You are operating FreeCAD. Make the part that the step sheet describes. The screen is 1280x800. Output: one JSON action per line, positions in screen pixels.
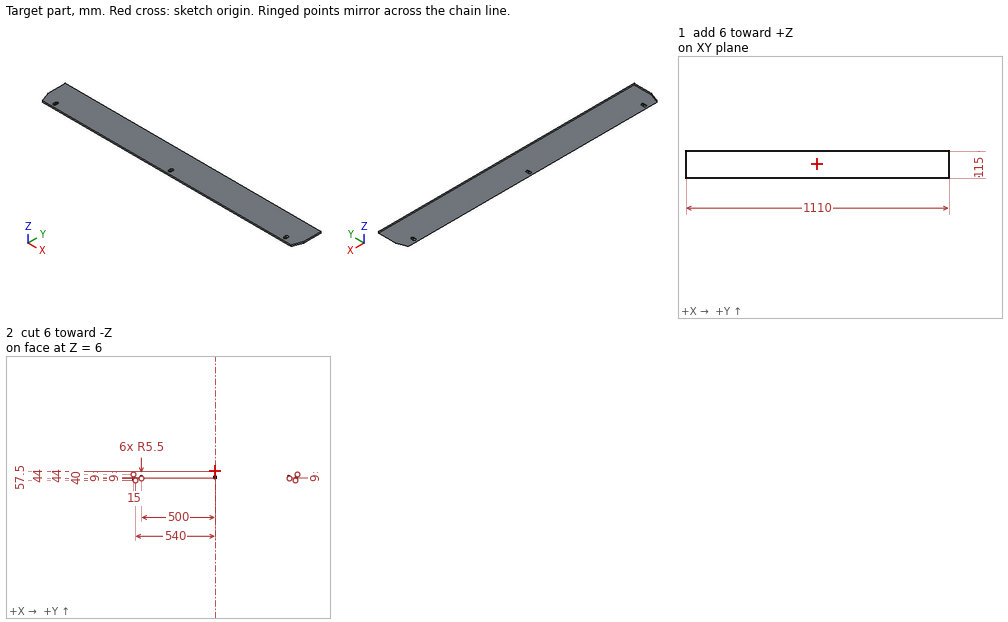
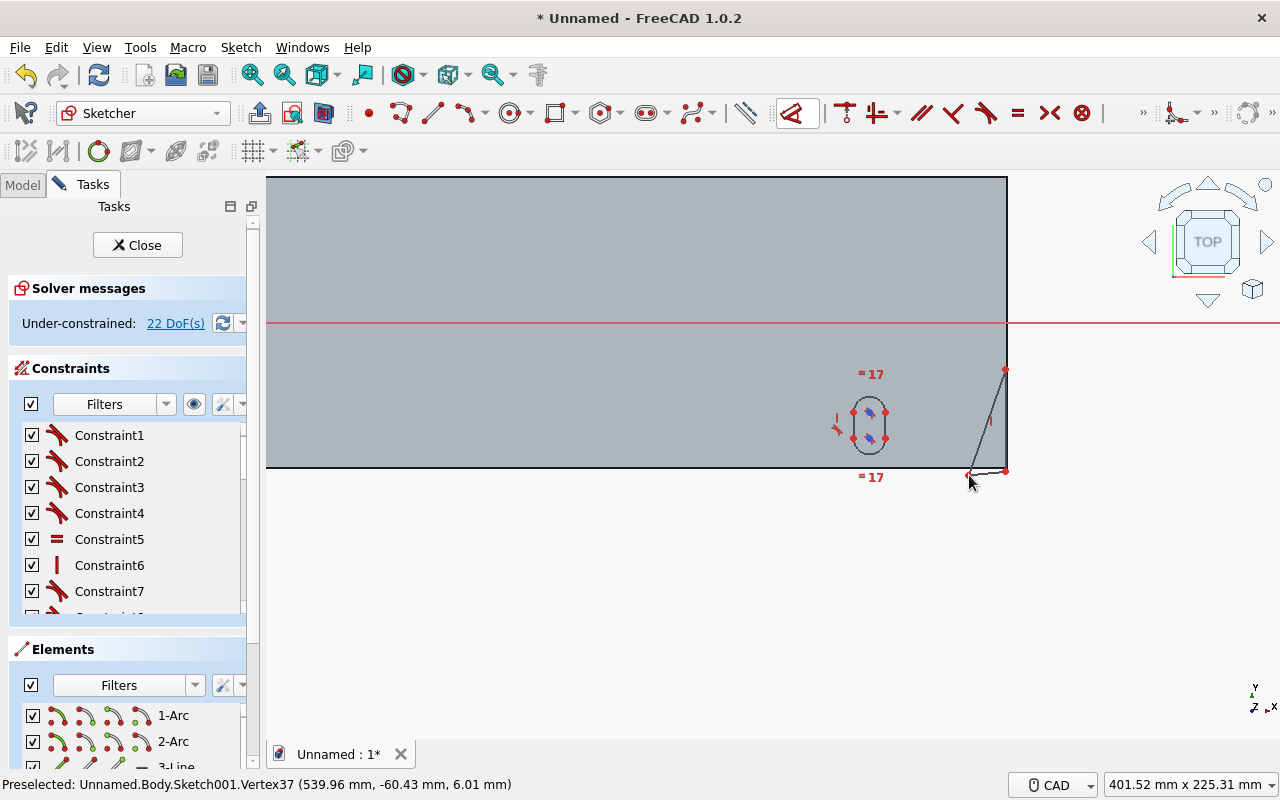
{"action": "scroll", "coordinate": [983, 469], "scroll_direction": "down", "scroll_amount": 8}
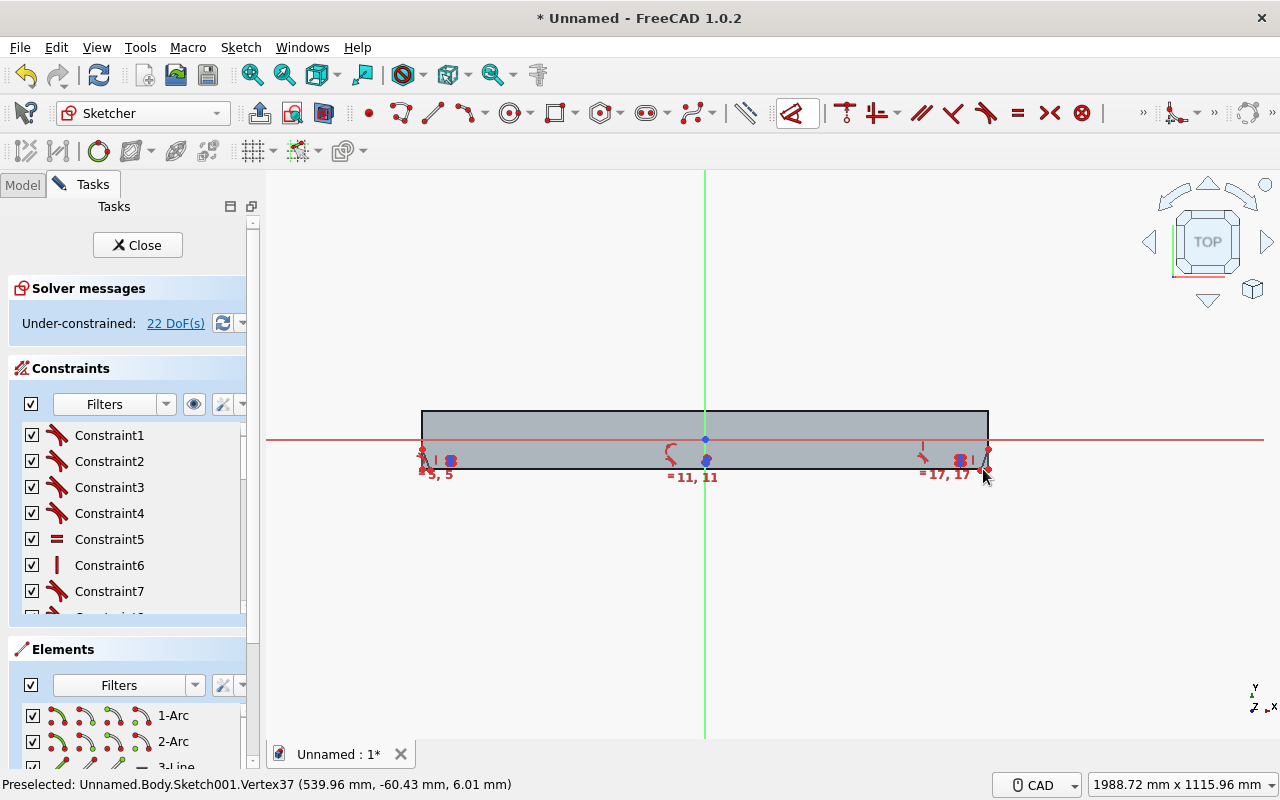
{"action": "scroll", "coordinate": [705, 461], "scroll_direction": "up", "scroll_amount": 9}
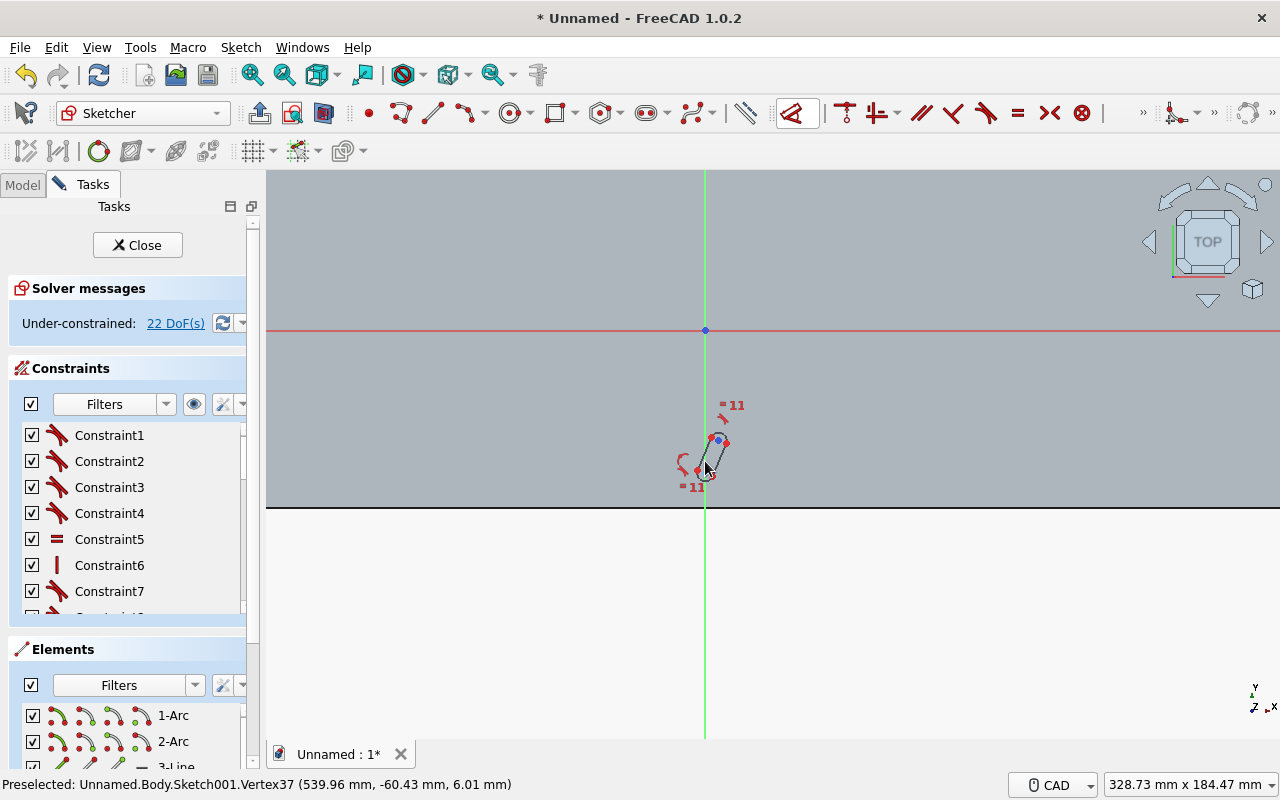
{"action": "left_click", "coordinate": [706, 451]}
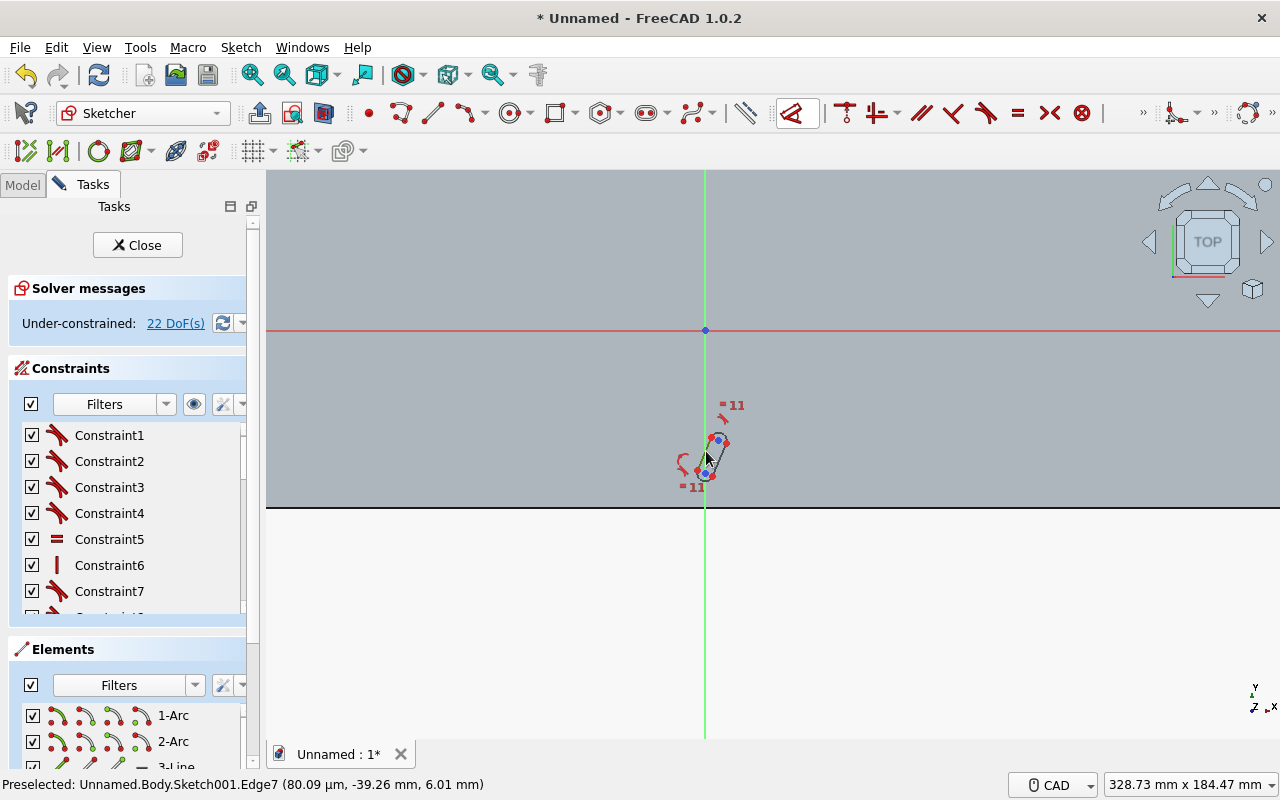
{"action": "left_click", "coordinate": [900, 114]}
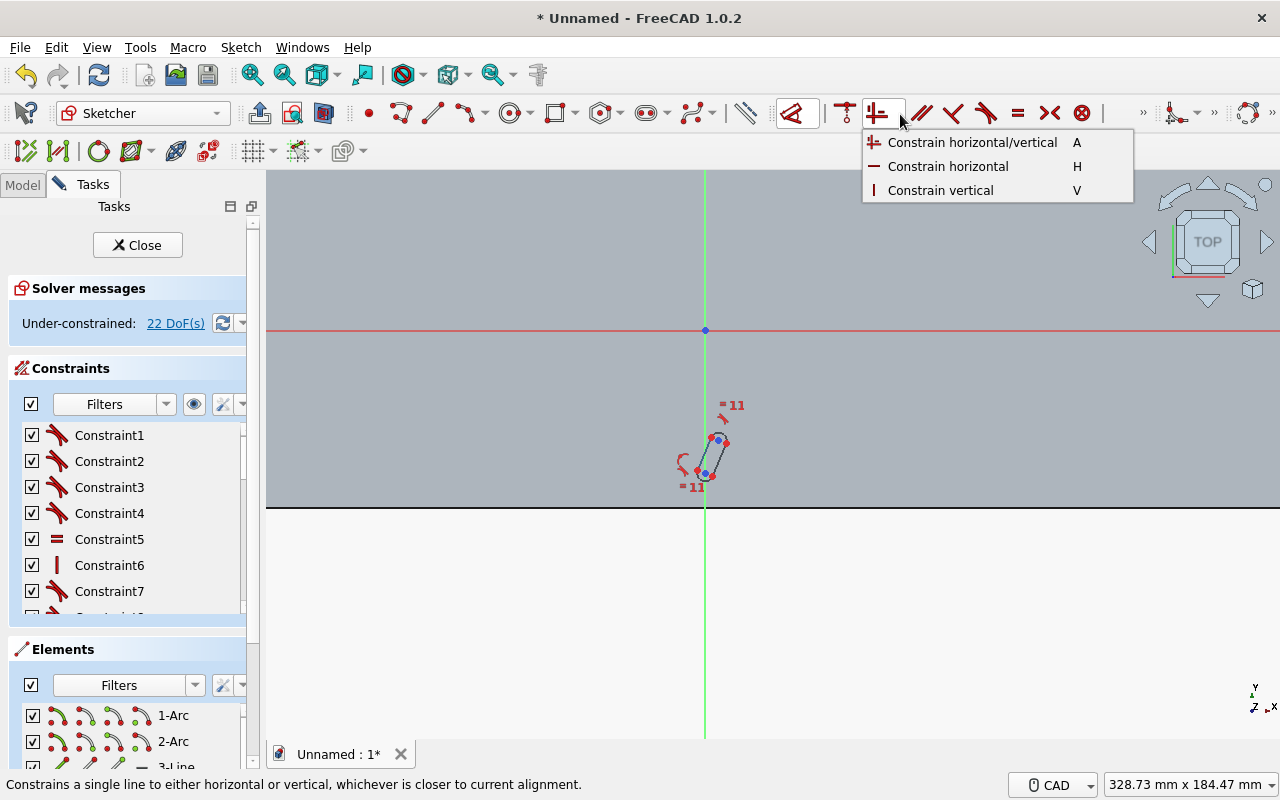
{"action": "left_click", "coordinate": [998, 190]}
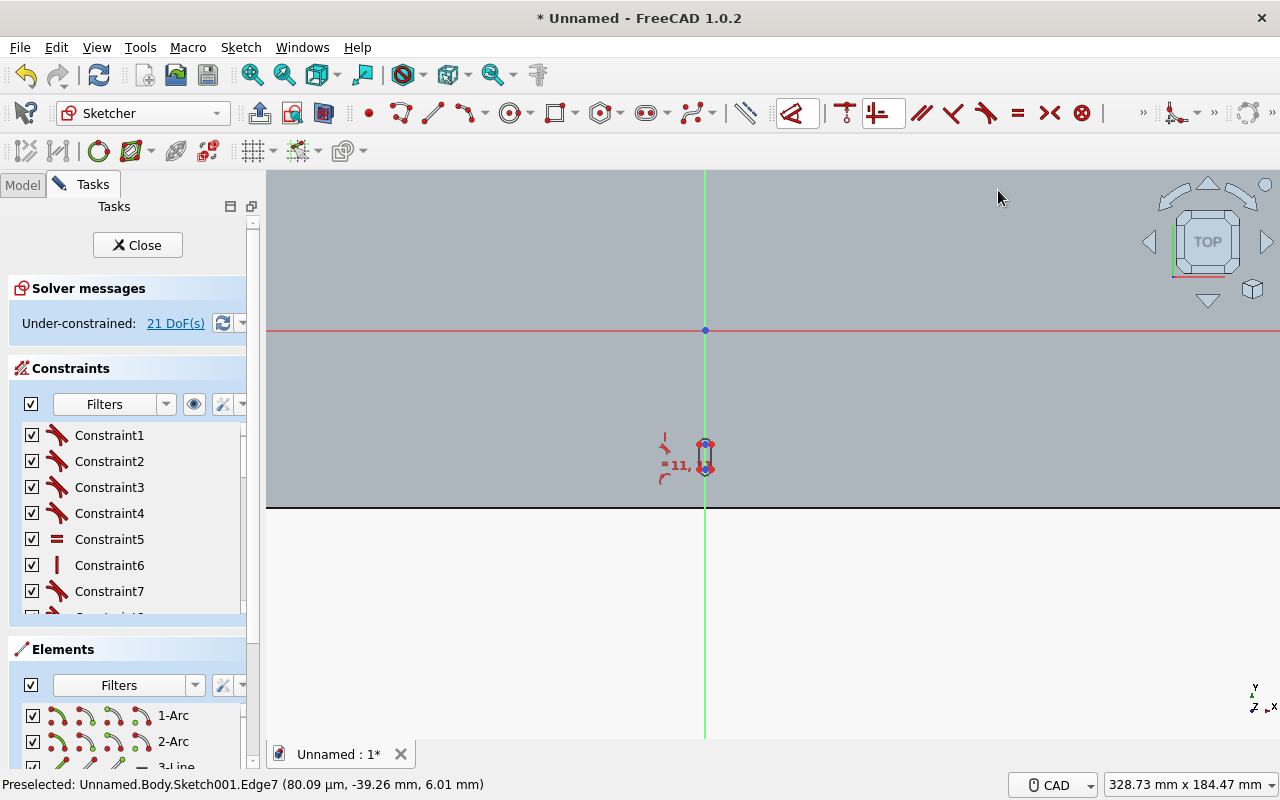
{"action": "scroll", "coordinate": [704, 461], "scroll_direction": "down", "scroll_amount": 9}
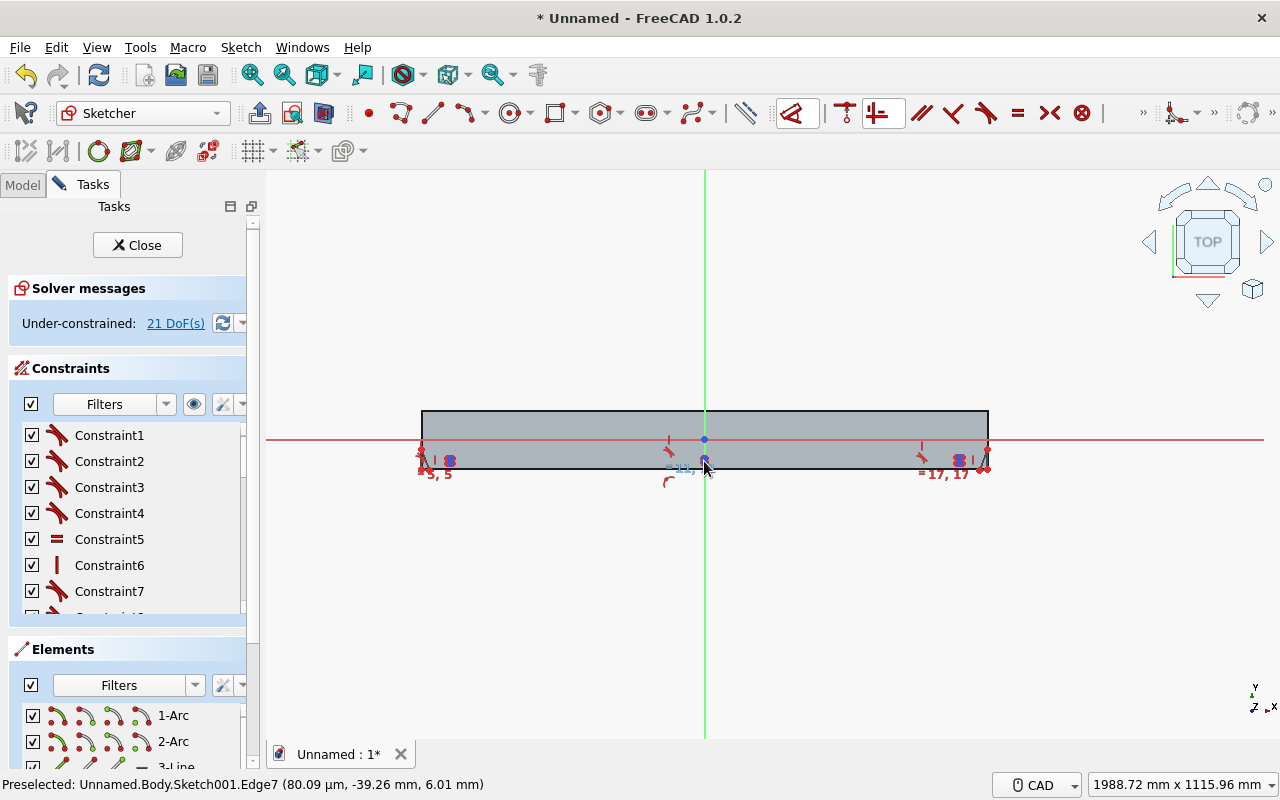
{"action": "scroll", "coordinate": [424, 470], "scroll_direction": "up", "scroll_amount": 9}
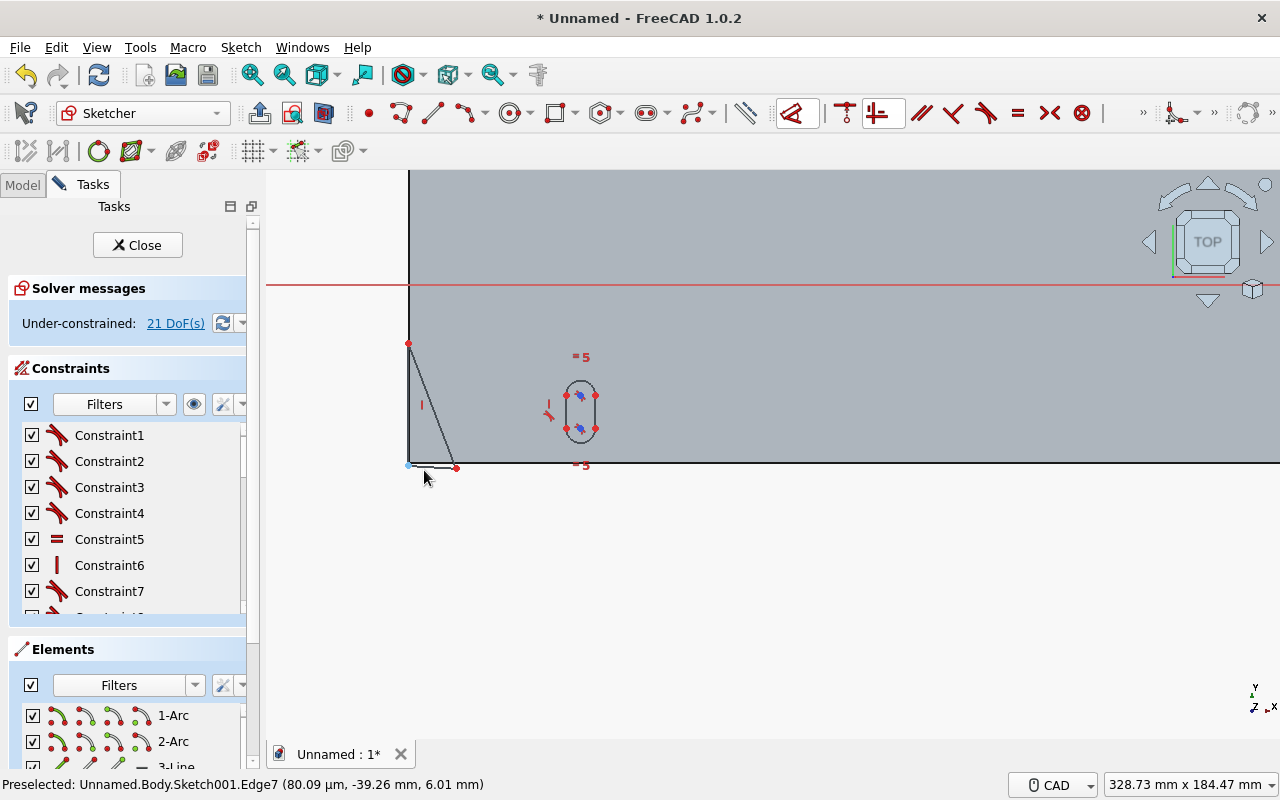
{"action": "left_click", "coordinate": [422, 467]}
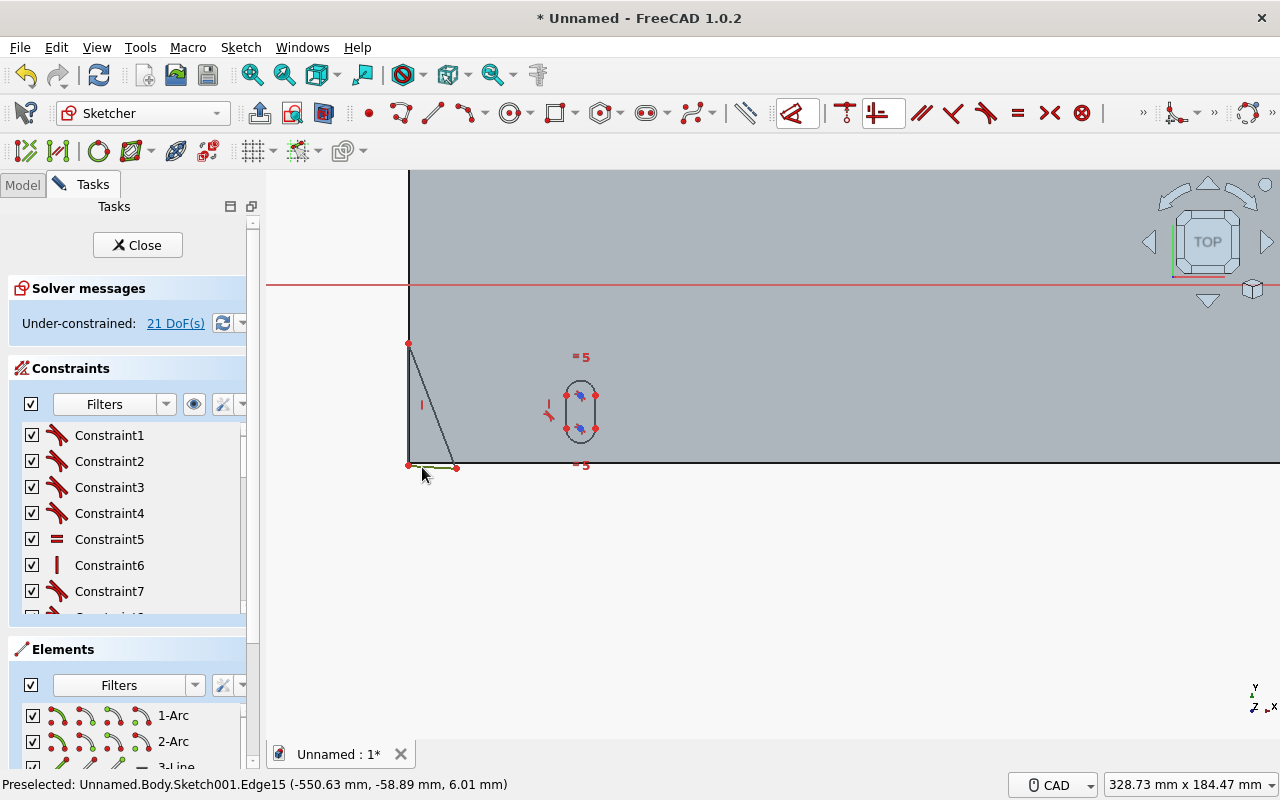
{"action": "key", "text": "h"}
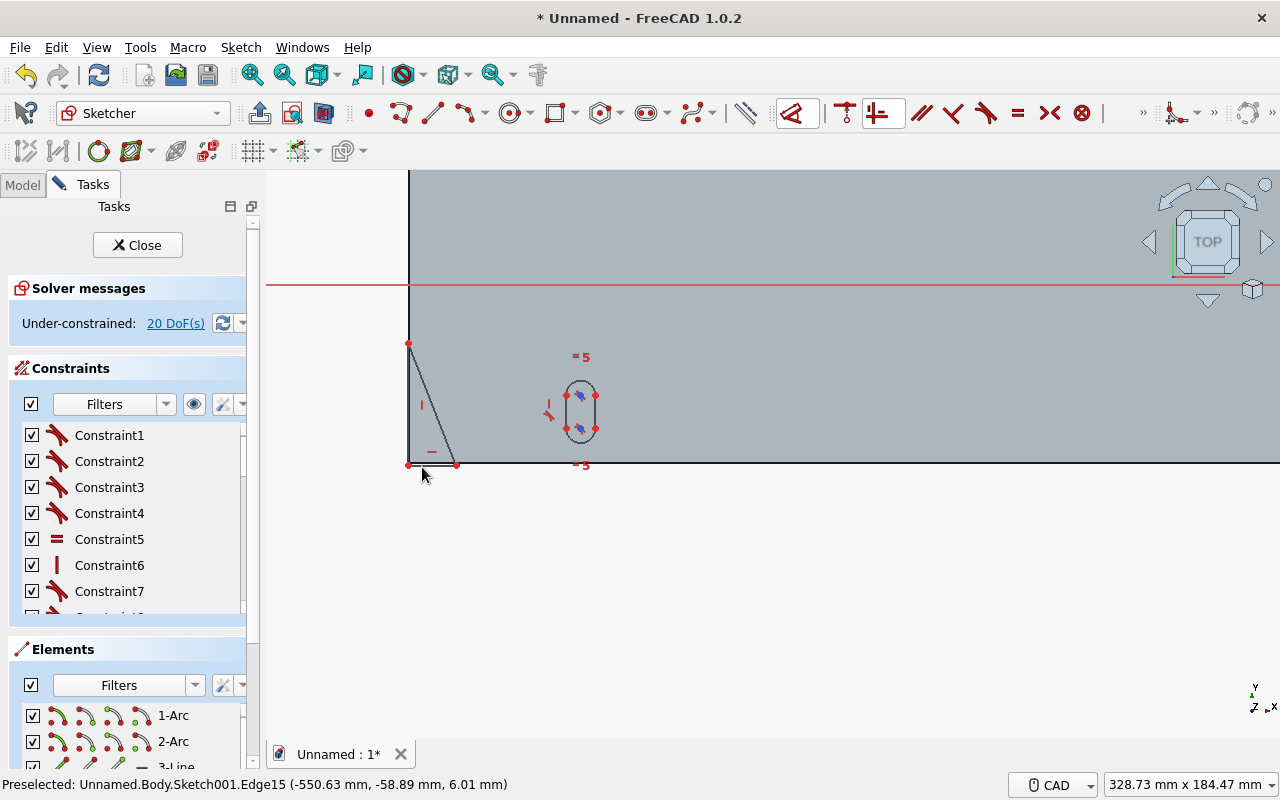
{"action": "scroll", "coordinate": [424, 470], "scroll_direction": "down", "scroll_amount": 9}